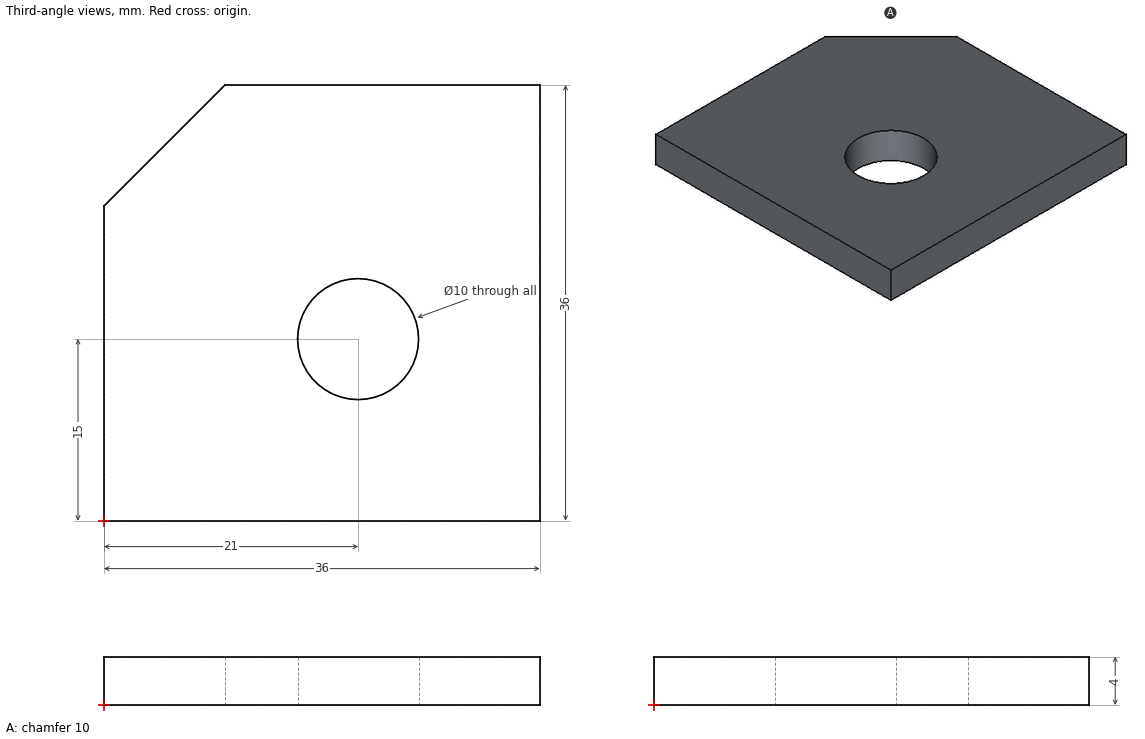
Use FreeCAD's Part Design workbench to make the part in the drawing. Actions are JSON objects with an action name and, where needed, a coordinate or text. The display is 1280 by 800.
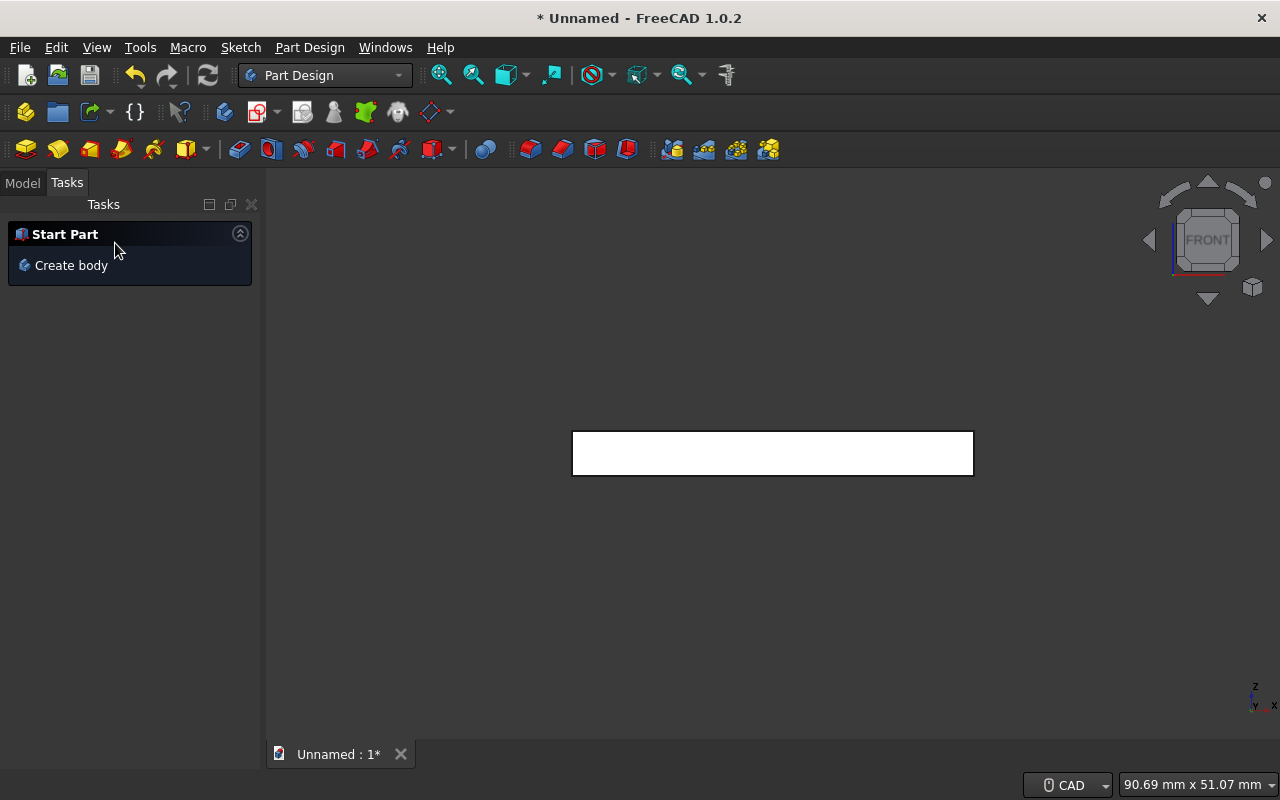
{"action": "key", "text": "v f"}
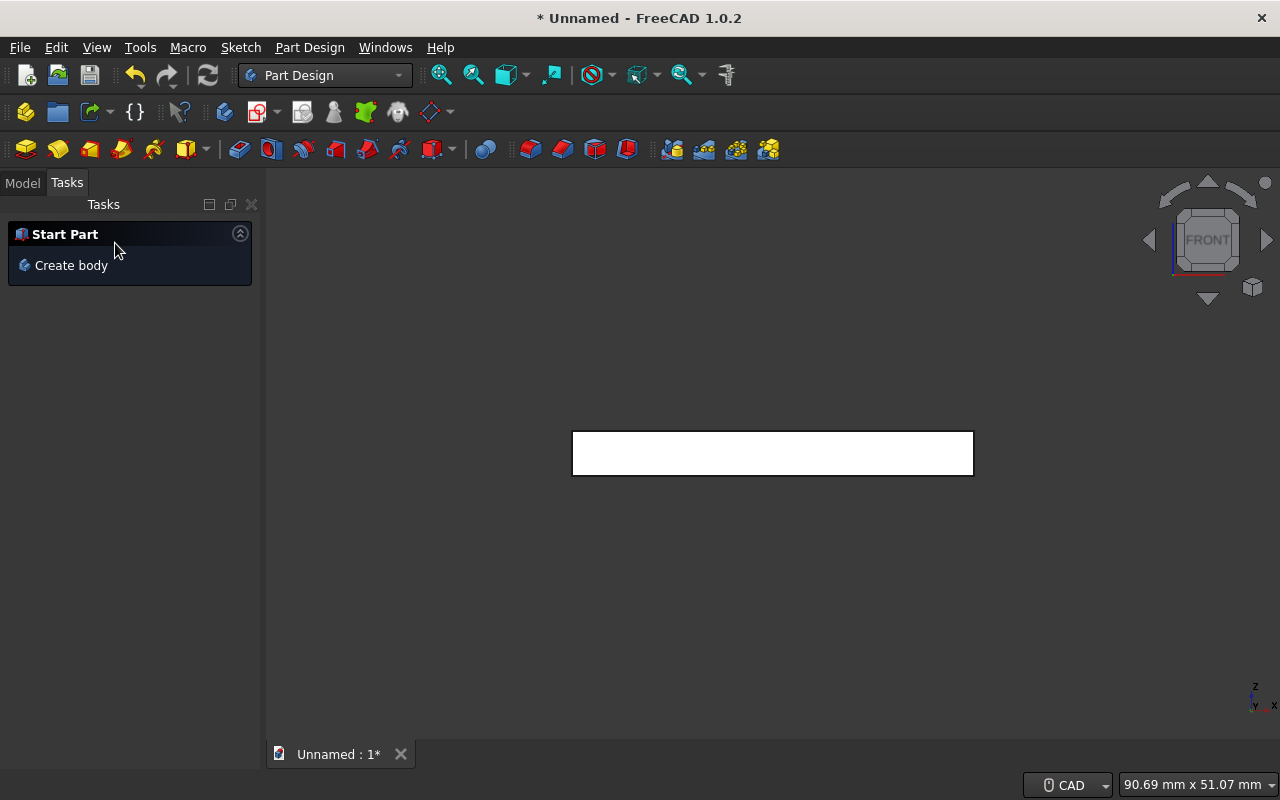
{"action": "key", "text": "3"}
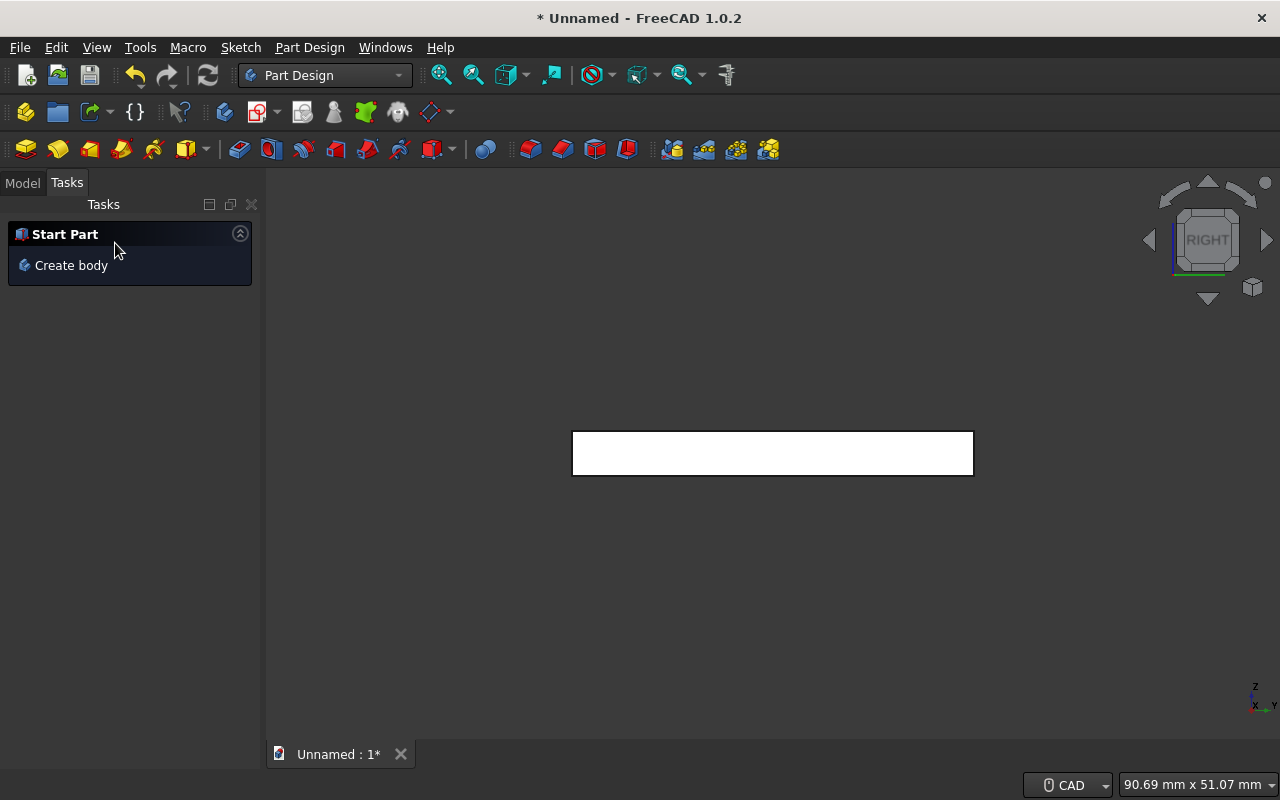
{"action": "key", "text": "v f"}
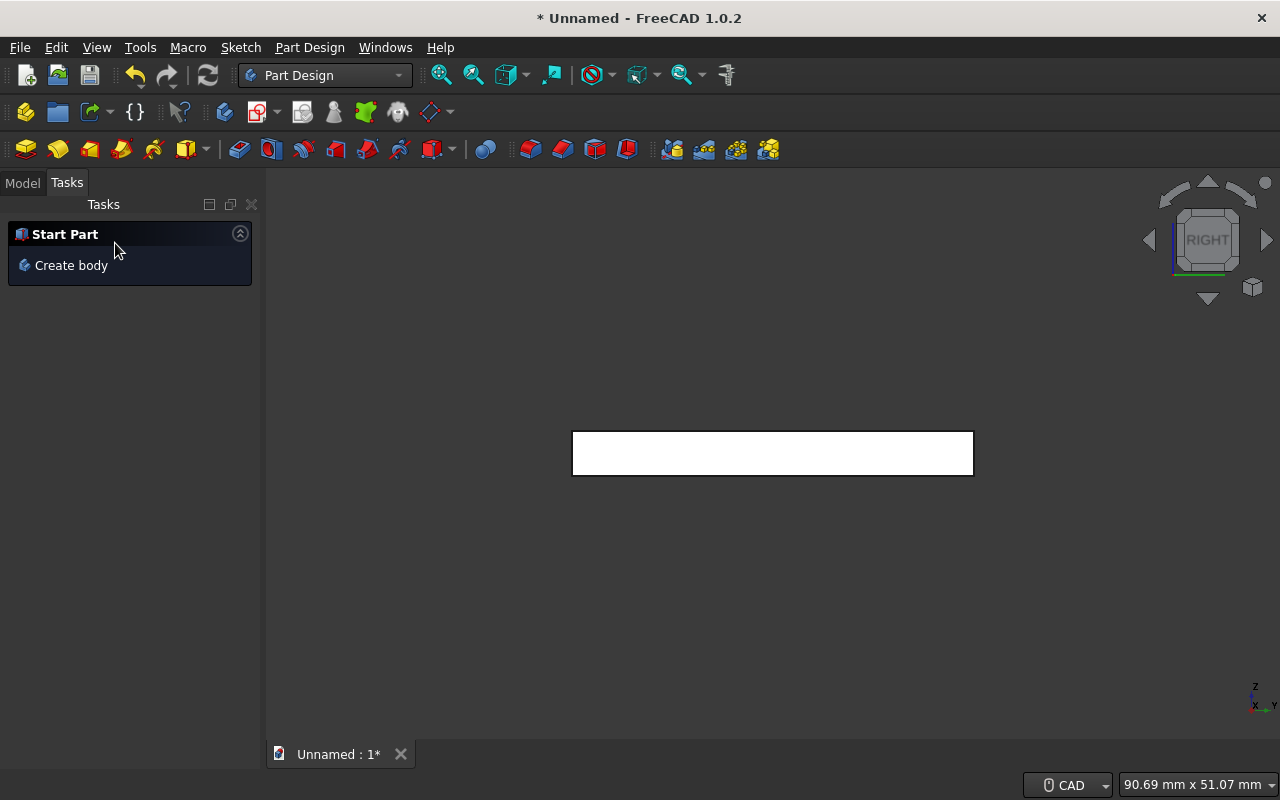
{"action": "key", "text": "5"}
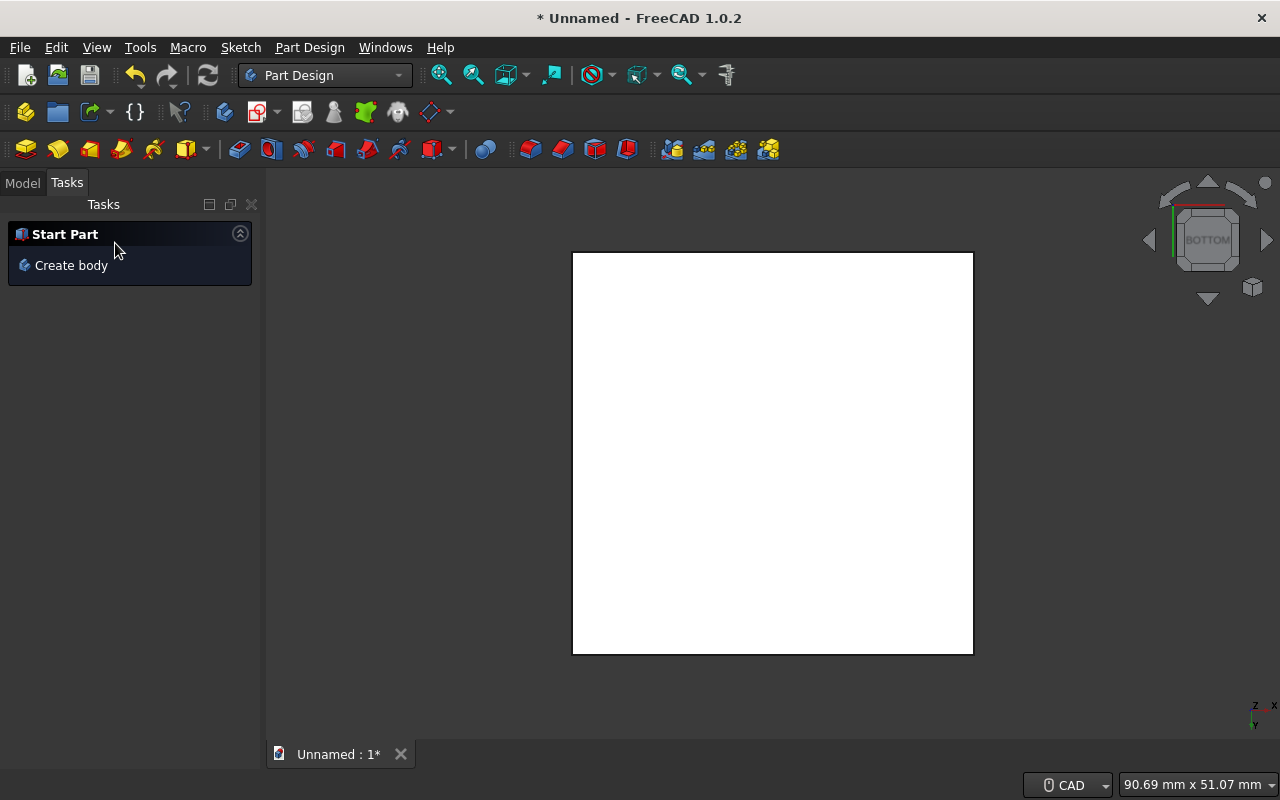
{"action": "key", "text": "4"}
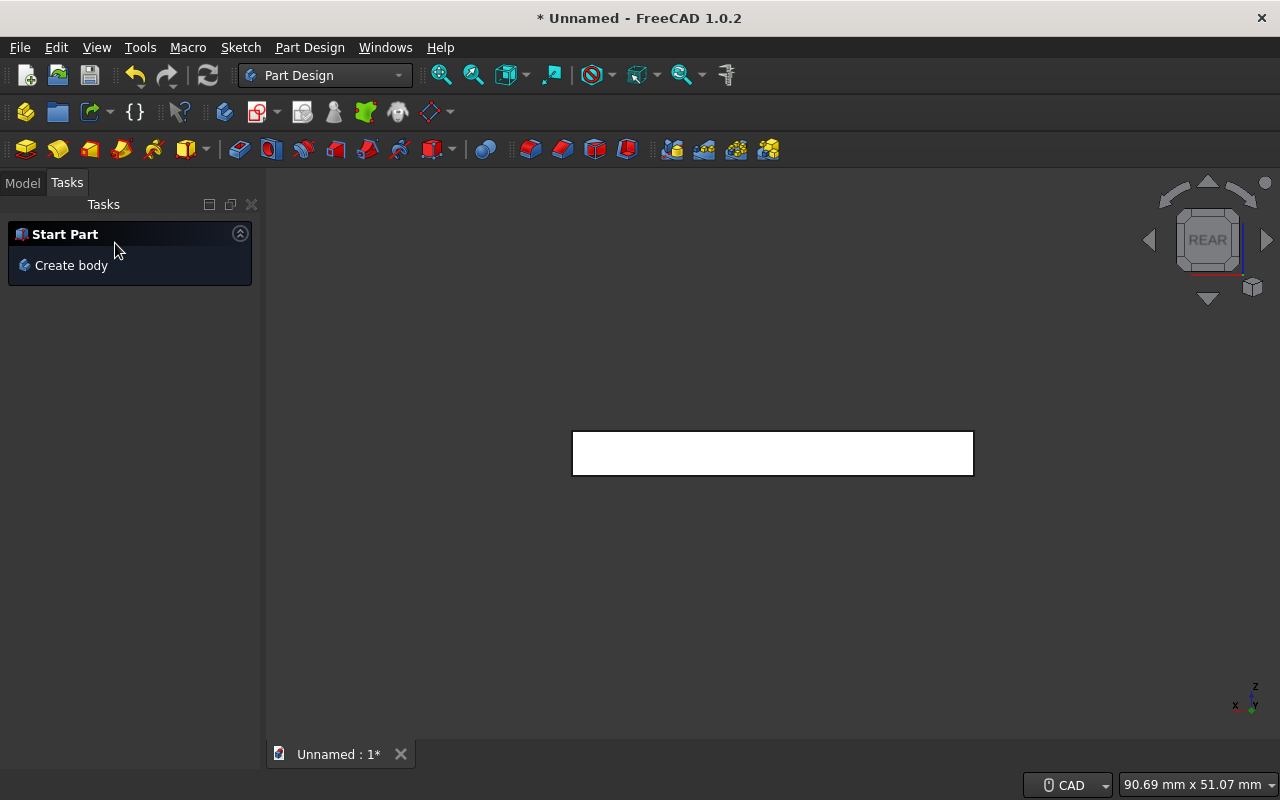
{"action": "key", "text": "v f"}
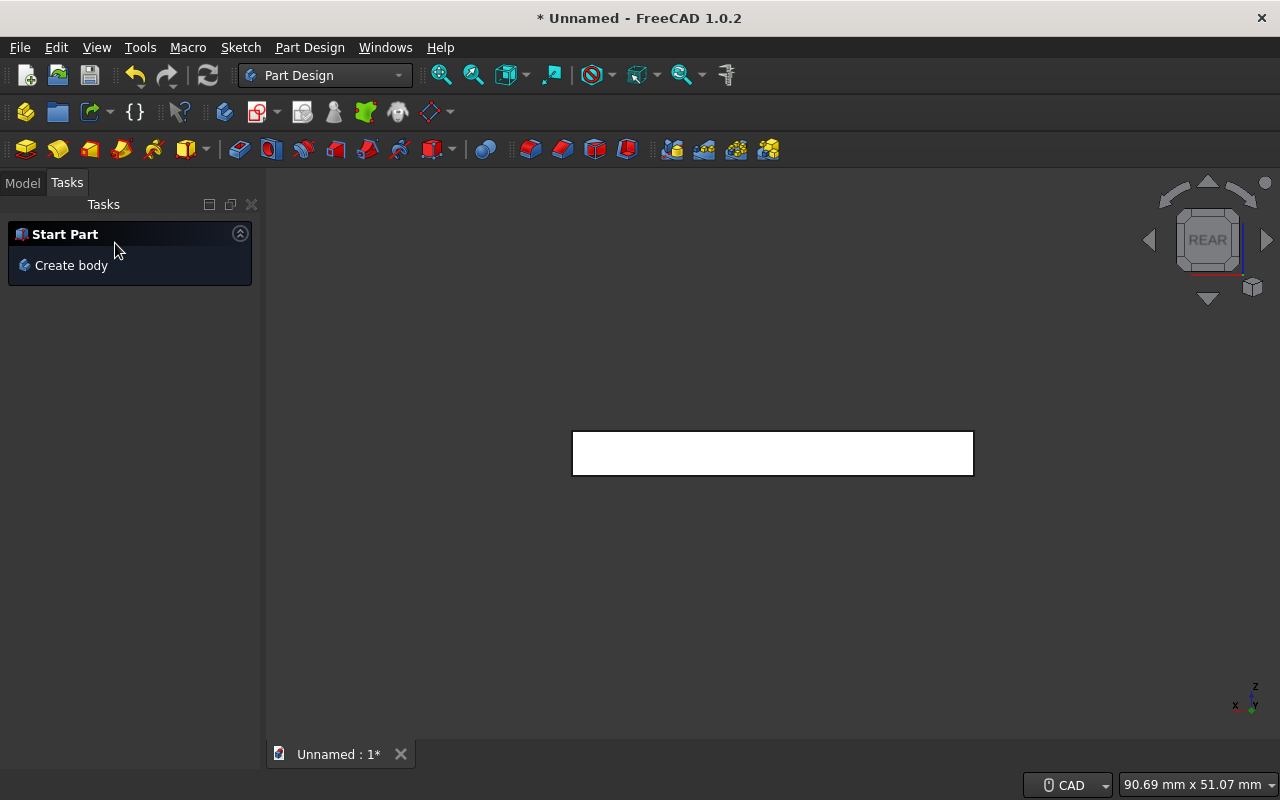
{"action": "left_click", "coordinate": [974, 453]}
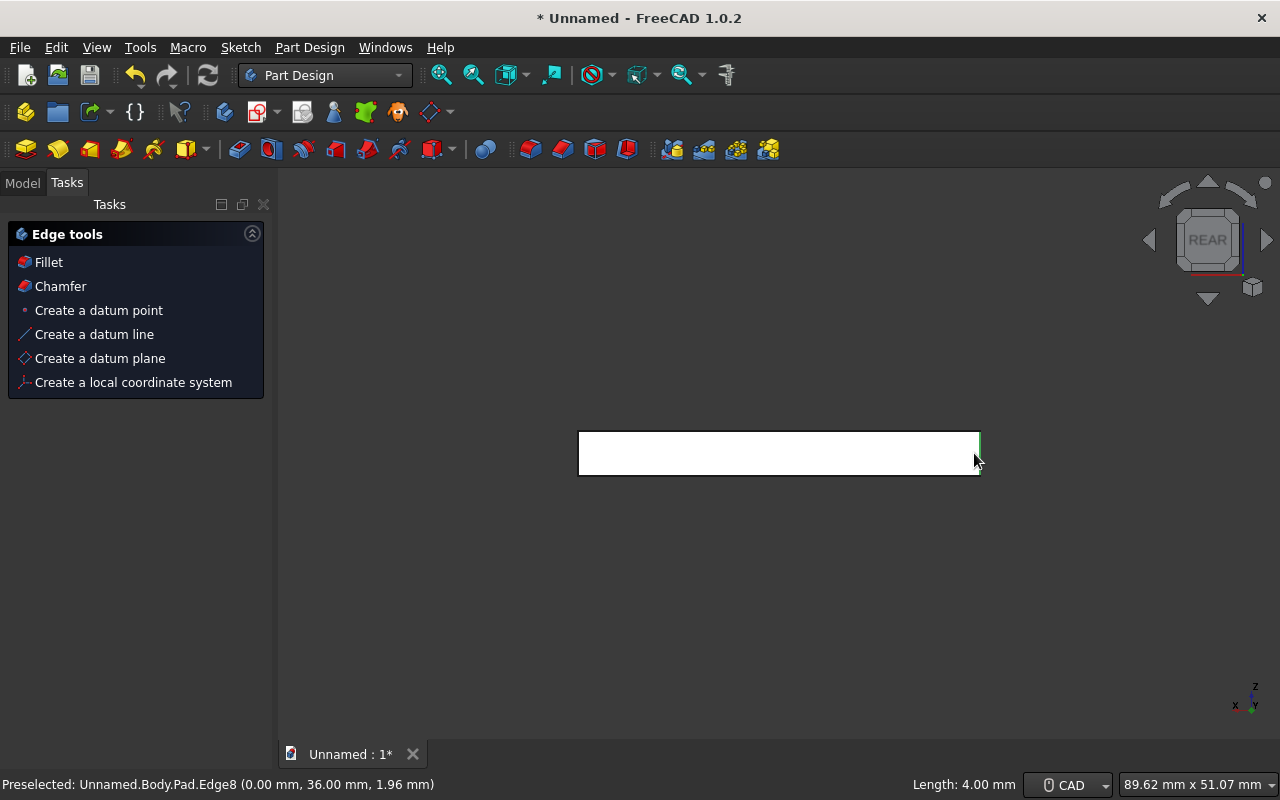
{"action": "left_click", "coordinate": [564, 150]}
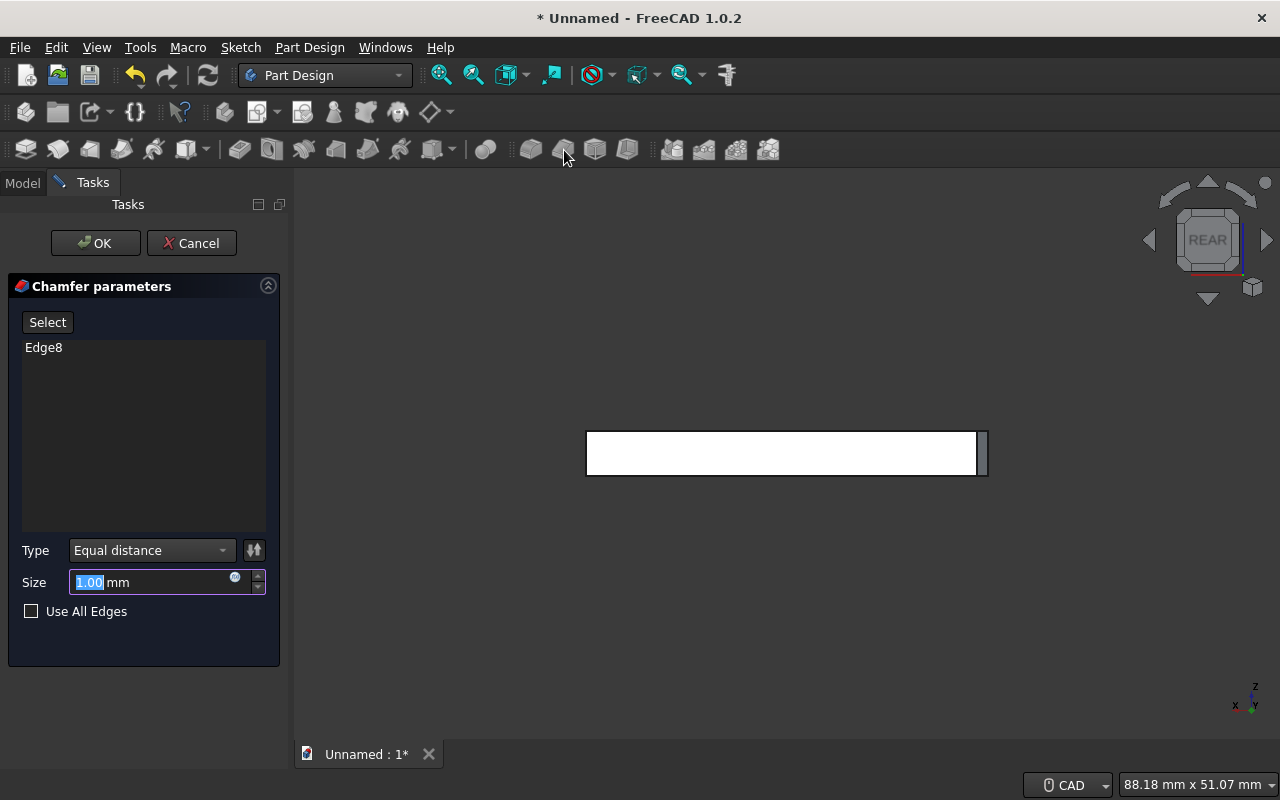
{"action": "type", "text": "10"}
{"action": "key", "text": "Tab"}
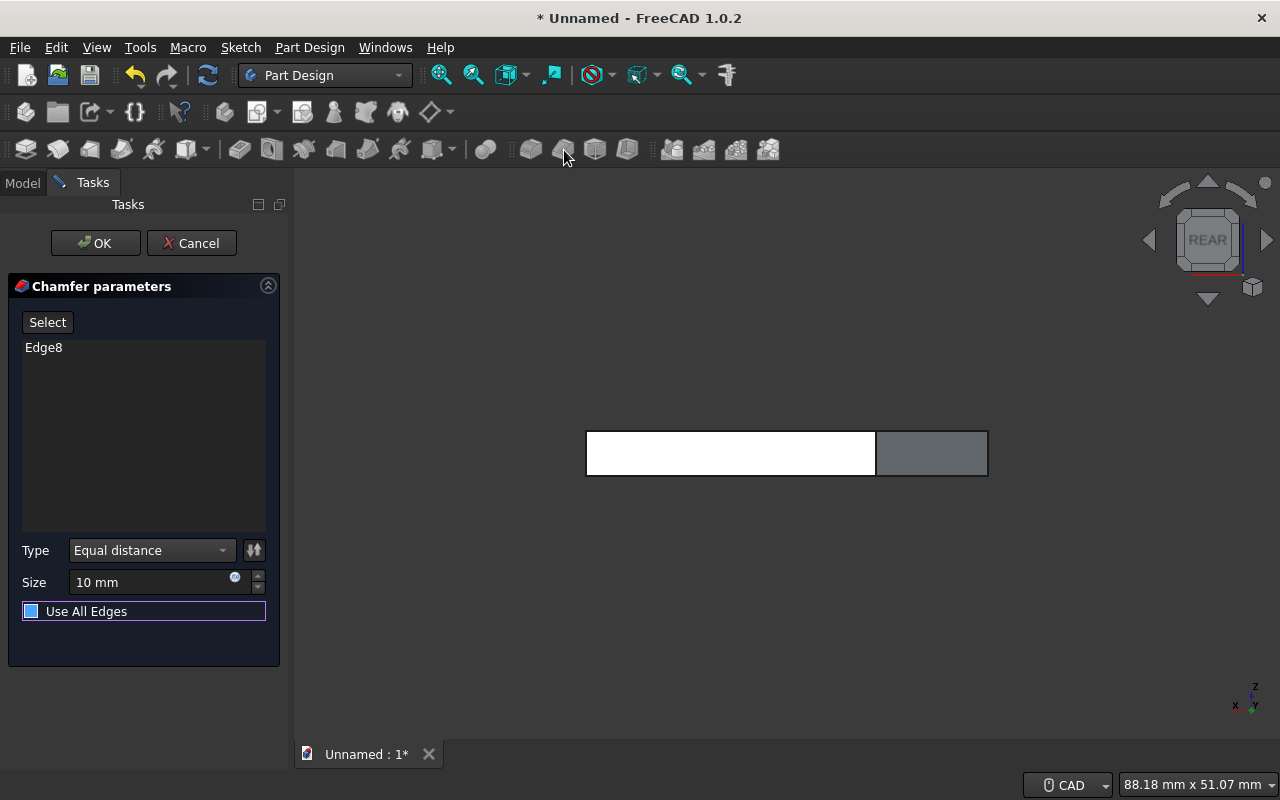
{"action": "left_click", "coordinate": [96, 243]}